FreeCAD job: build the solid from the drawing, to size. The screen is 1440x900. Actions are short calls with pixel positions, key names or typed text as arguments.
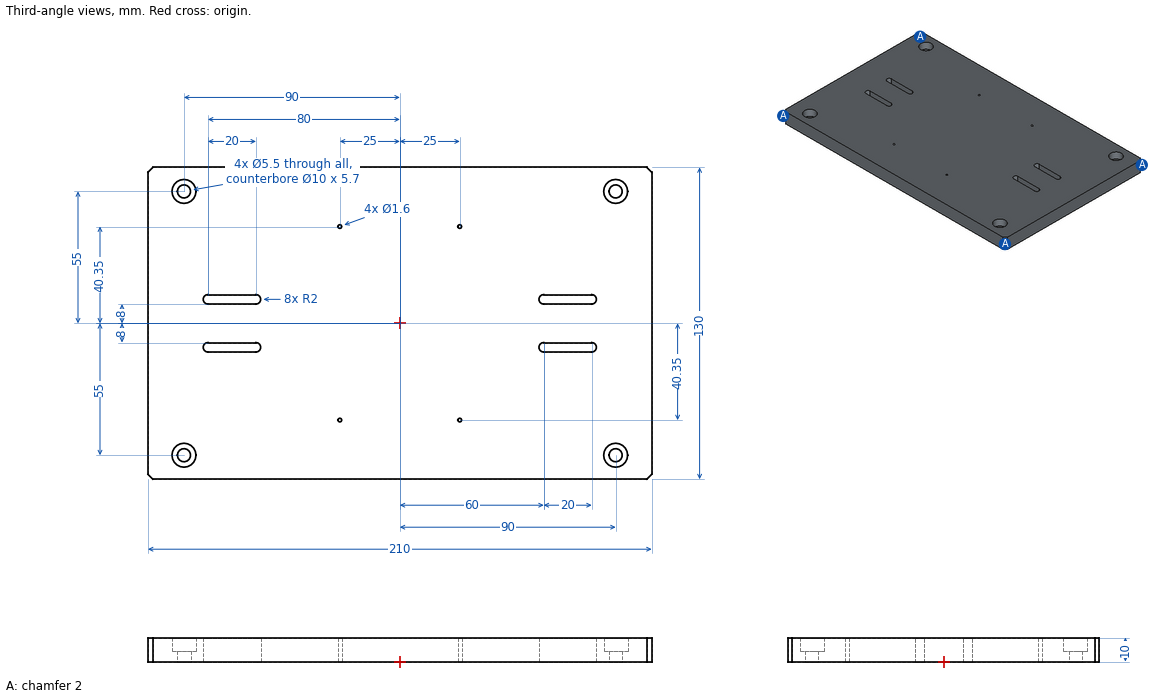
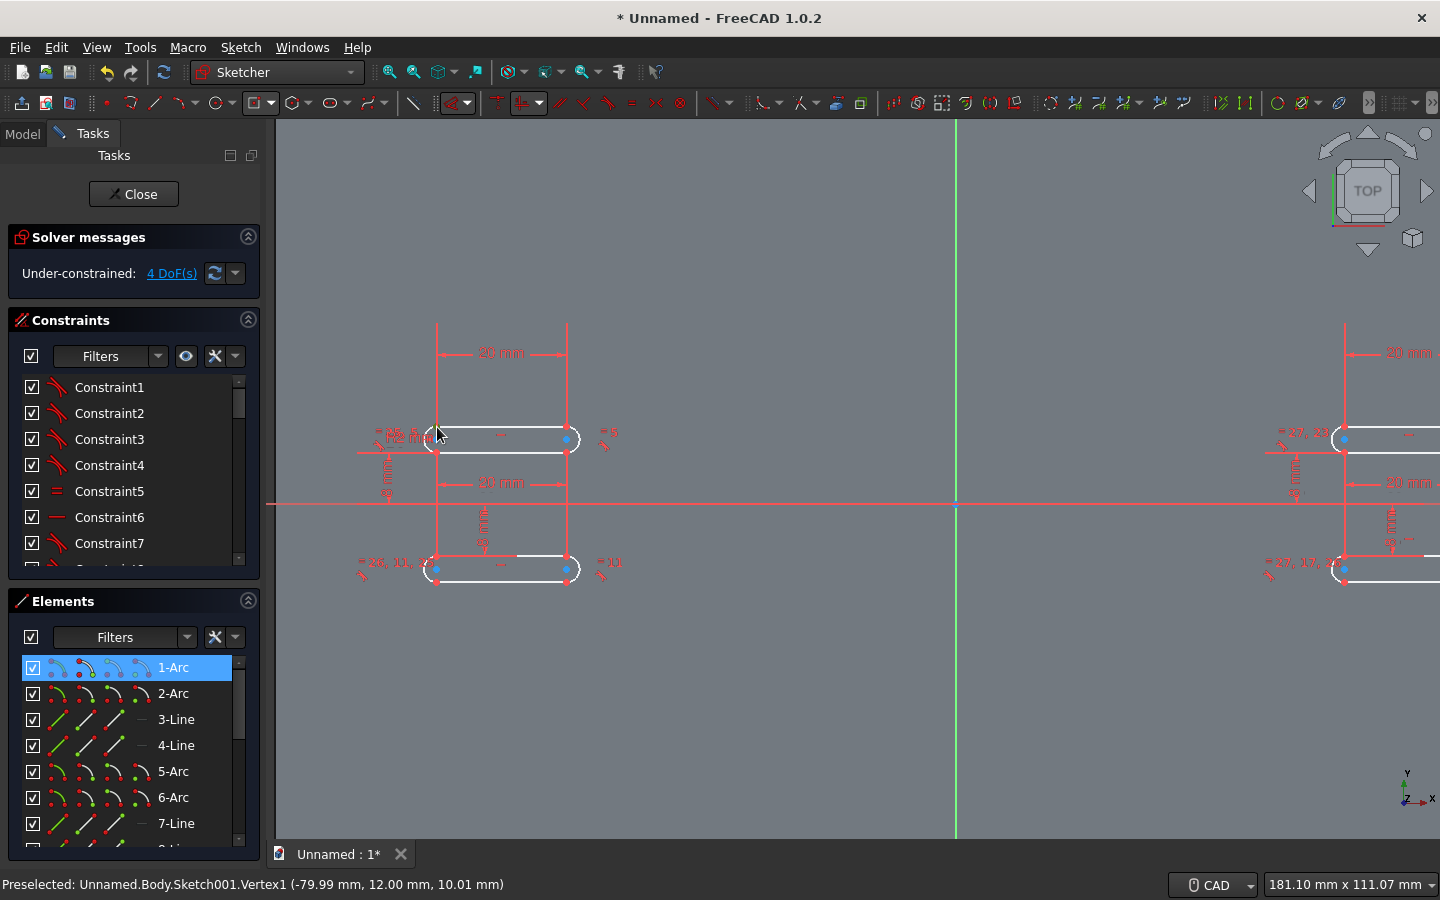
key(l)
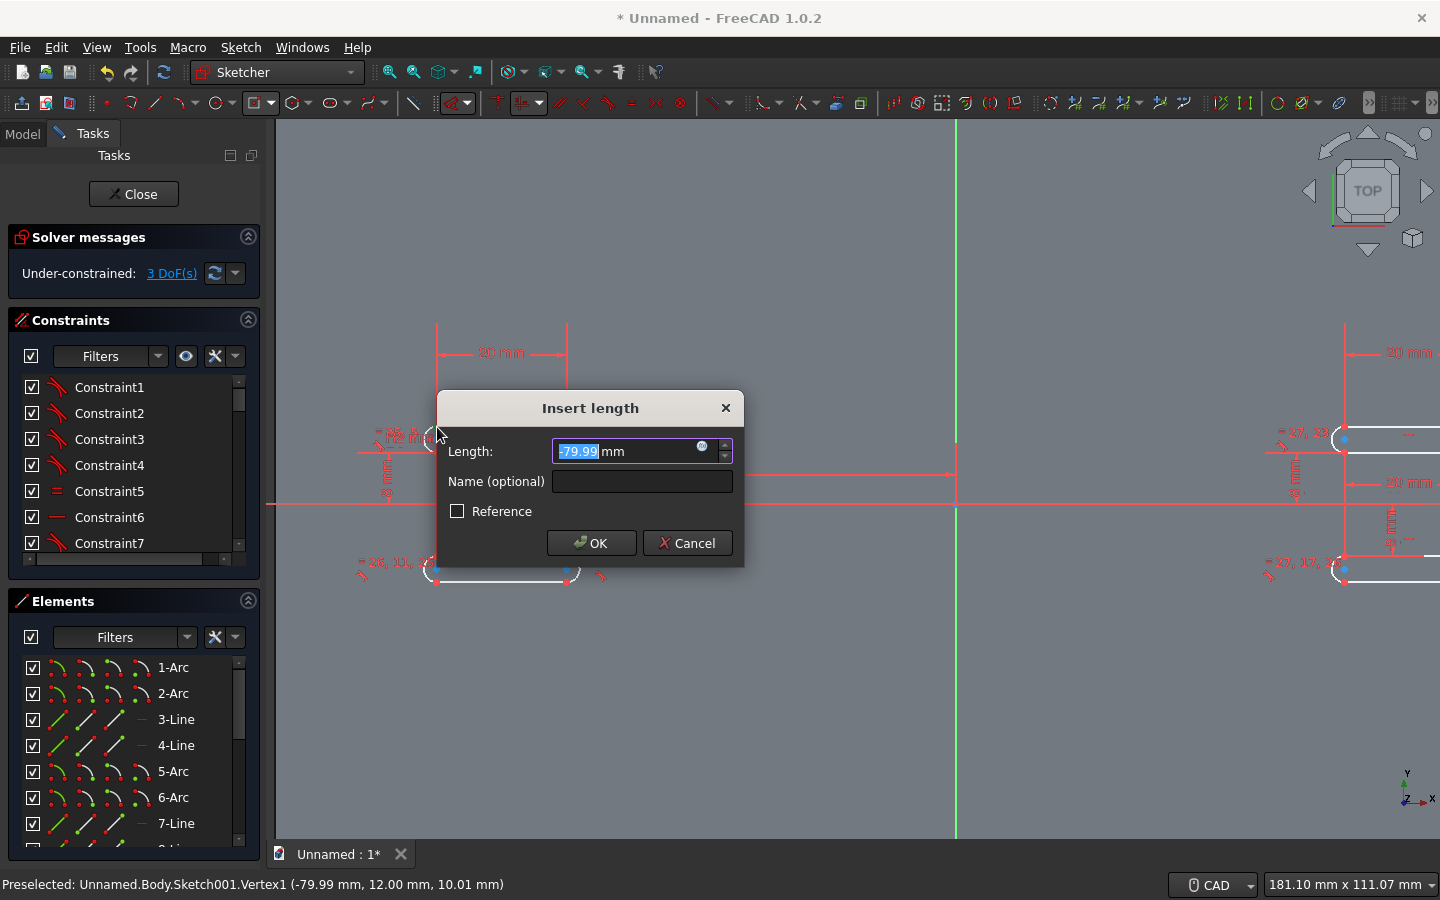
text(-80)
key(Return)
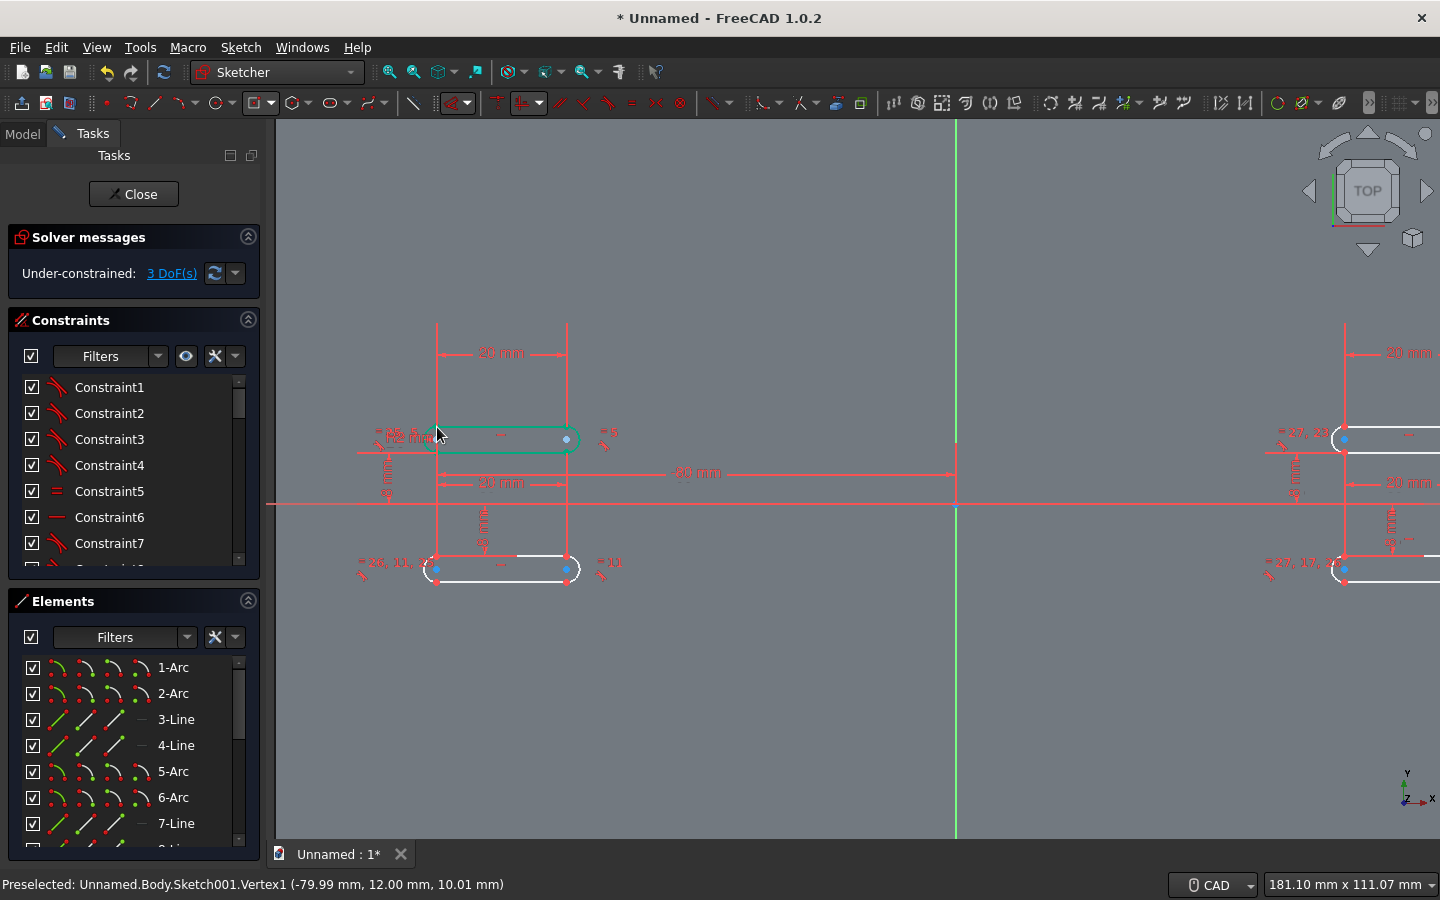
click(437, 556)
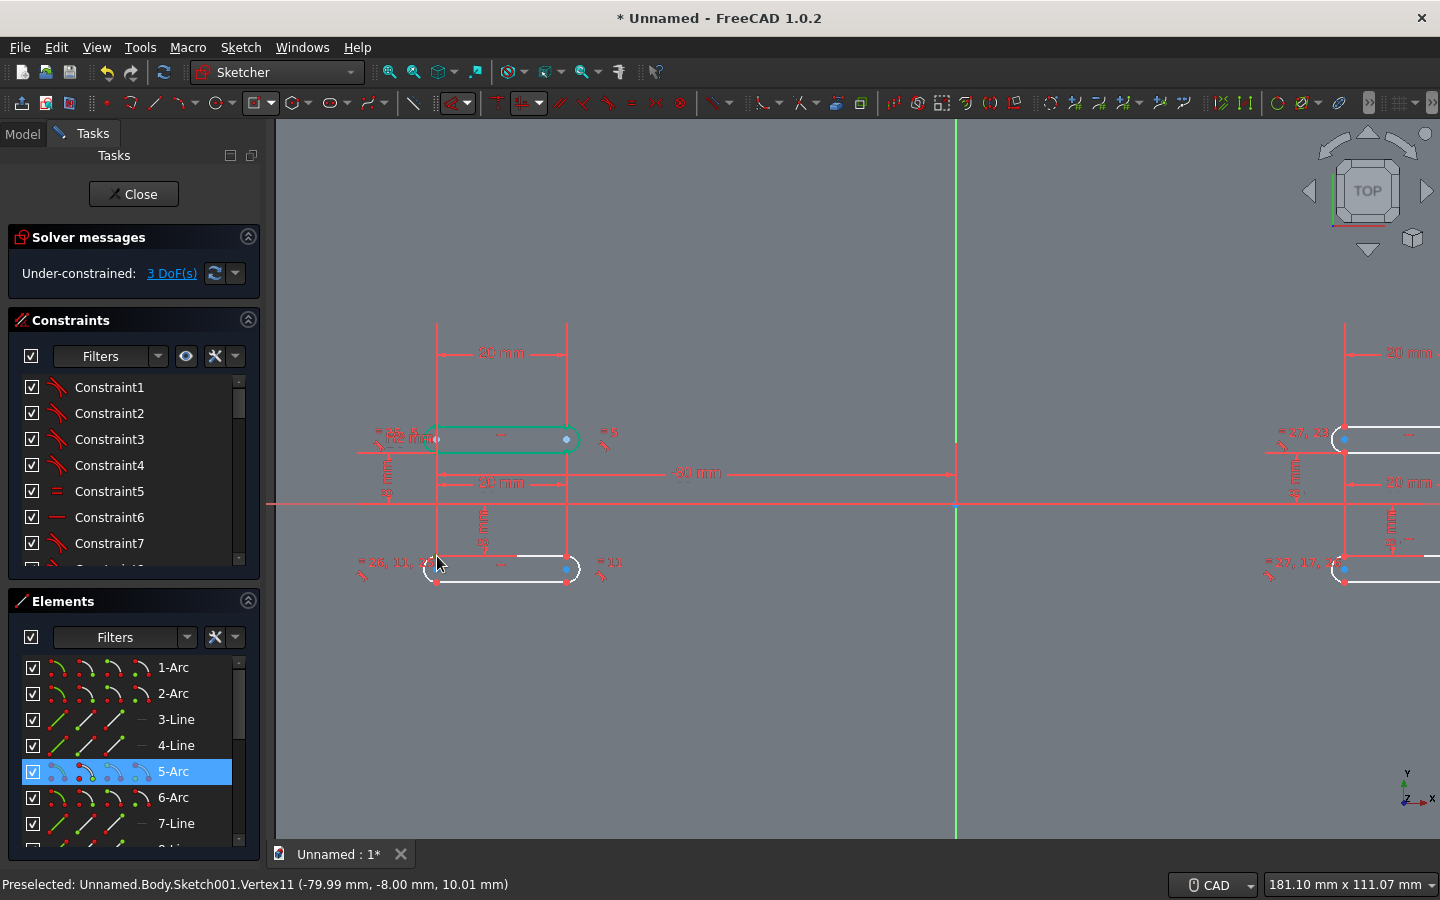
key(l)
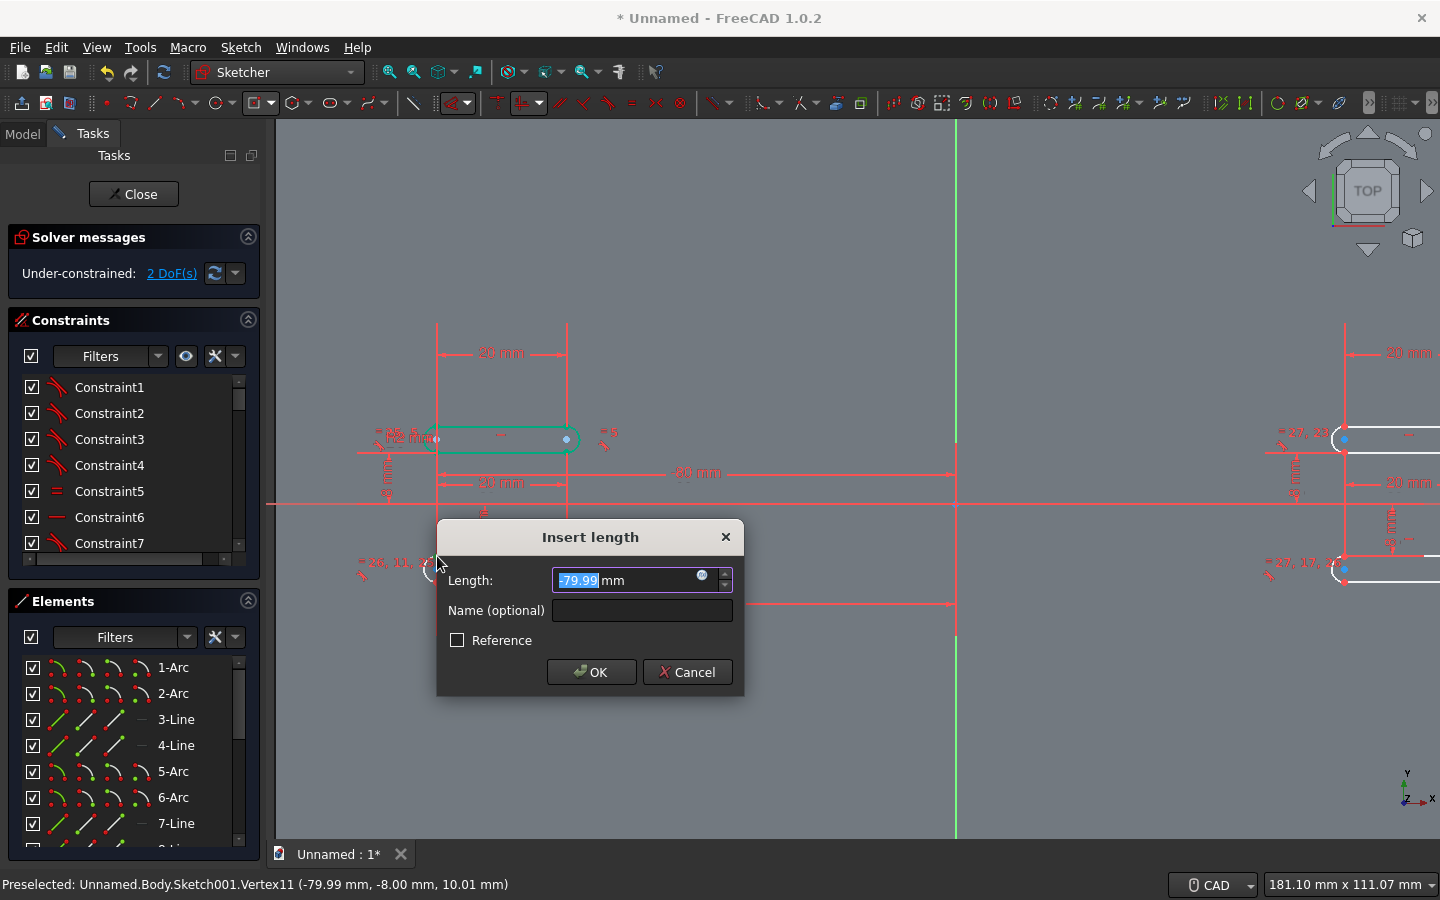
text(-80)
key(Return)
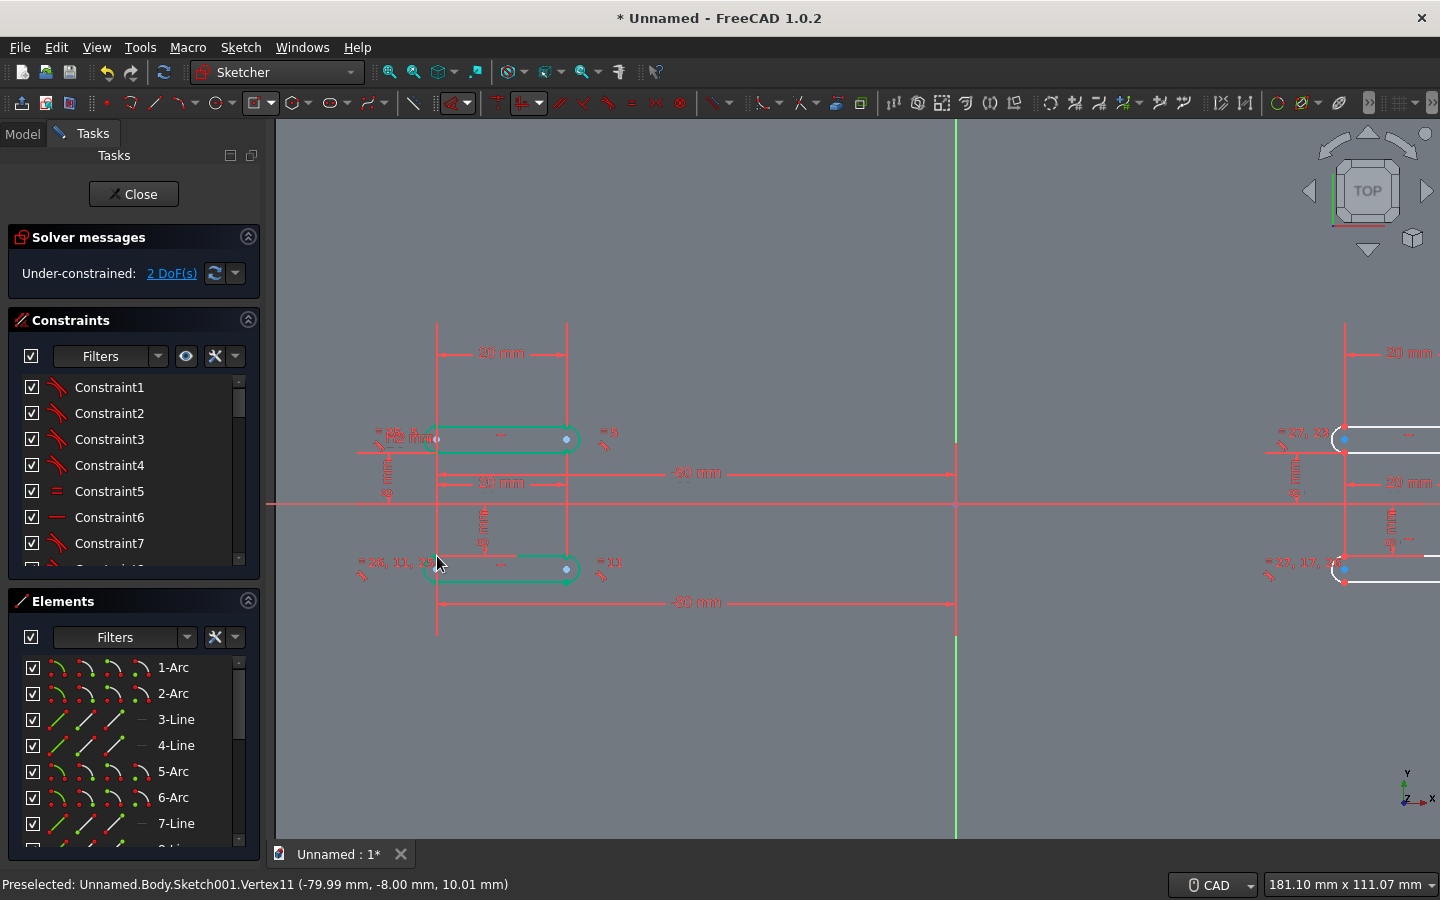
scroll(437, 427, down, 2)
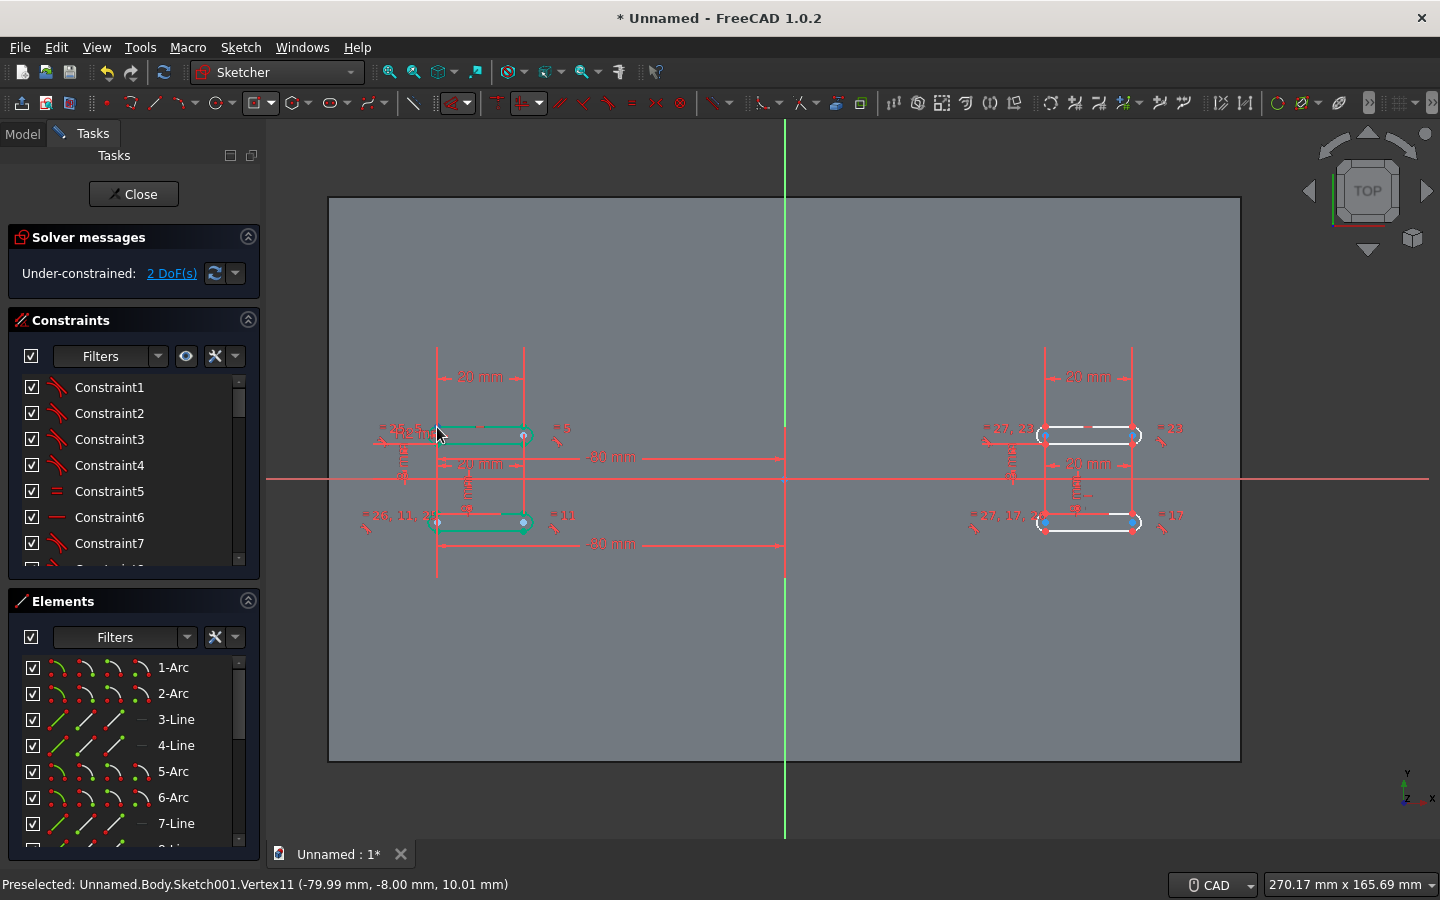
scroll(1045, 514, up, 2)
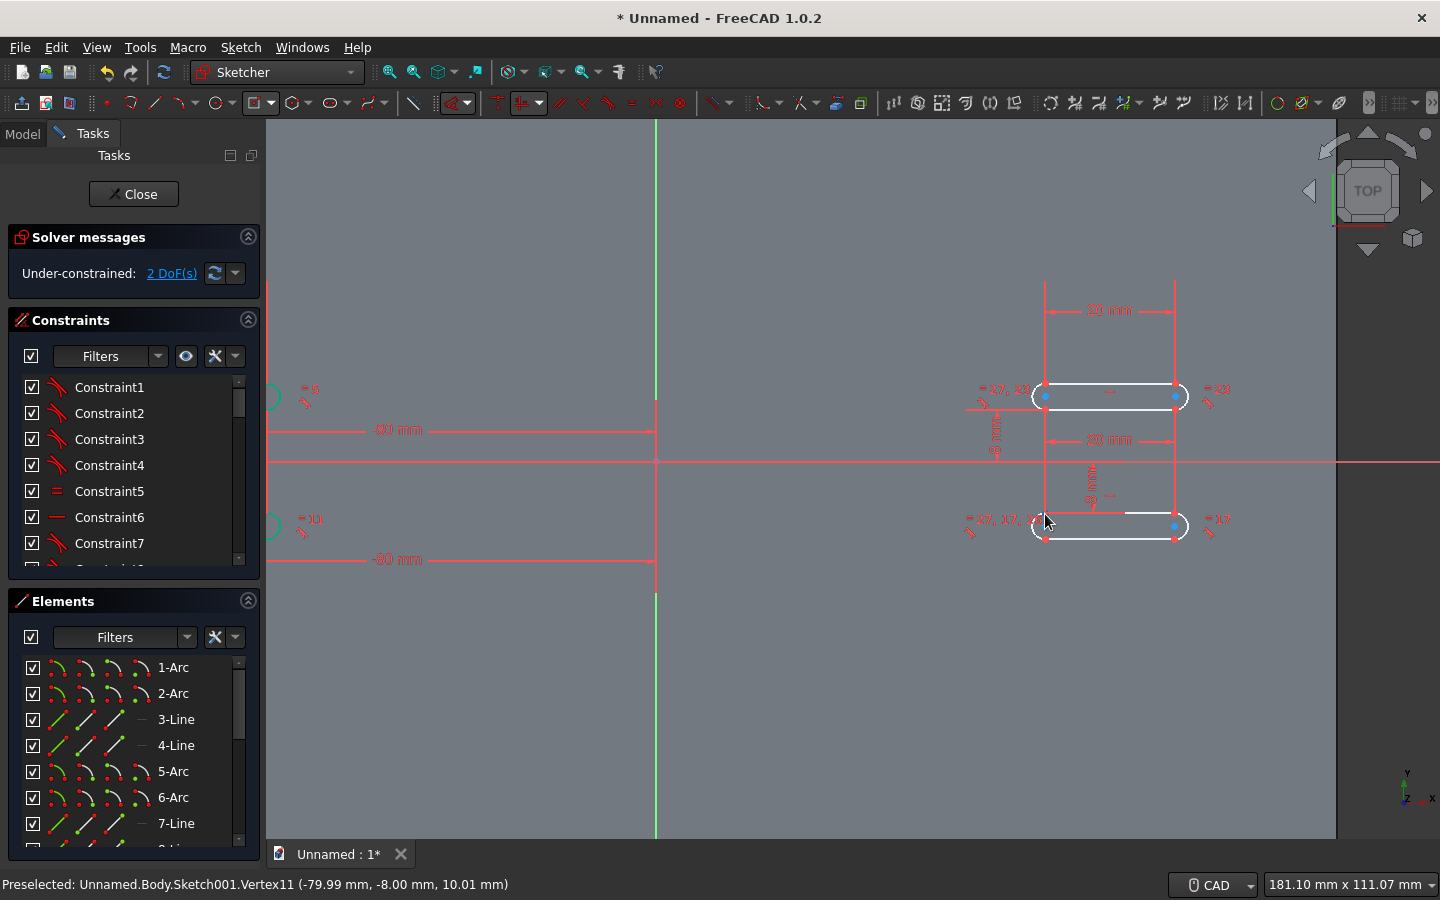
click(1045, 513)